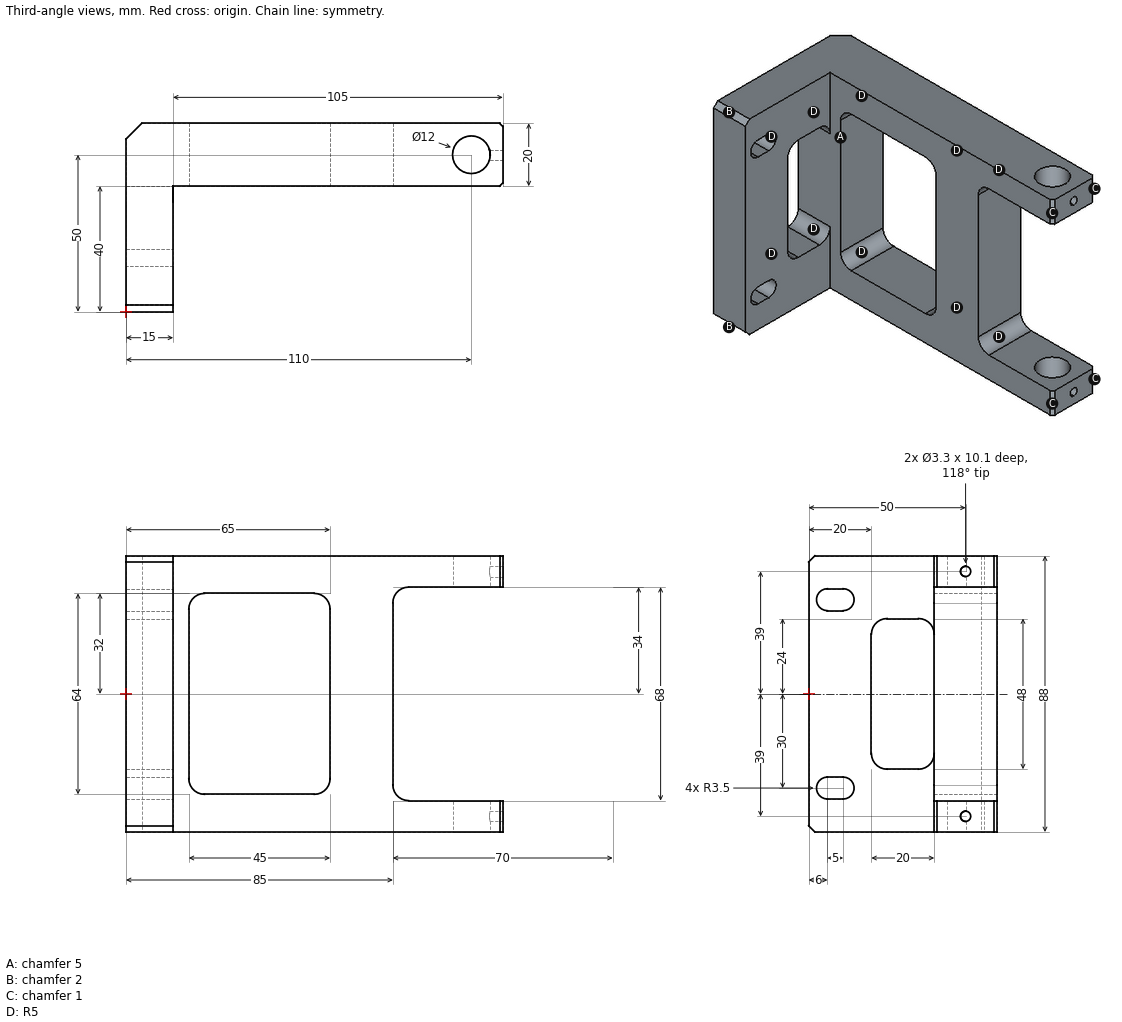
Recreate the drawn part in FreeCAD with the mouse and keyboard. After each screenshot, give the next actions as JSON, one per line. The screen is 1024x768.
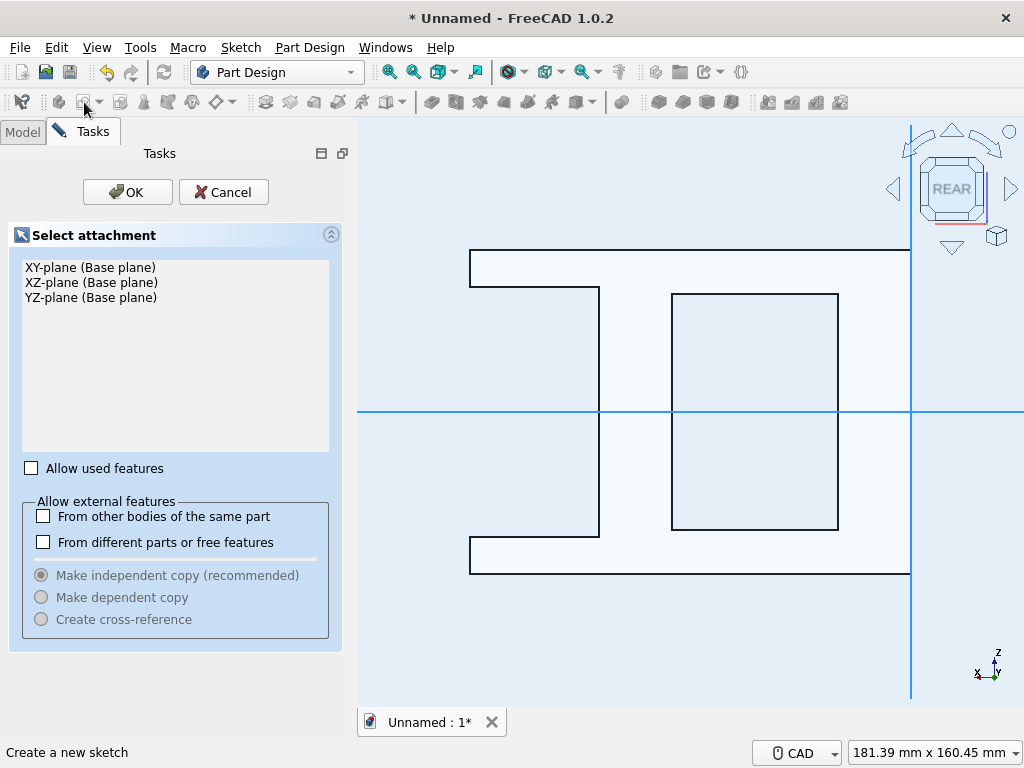
{"action": "left_click", "coordinate": [82, 298]}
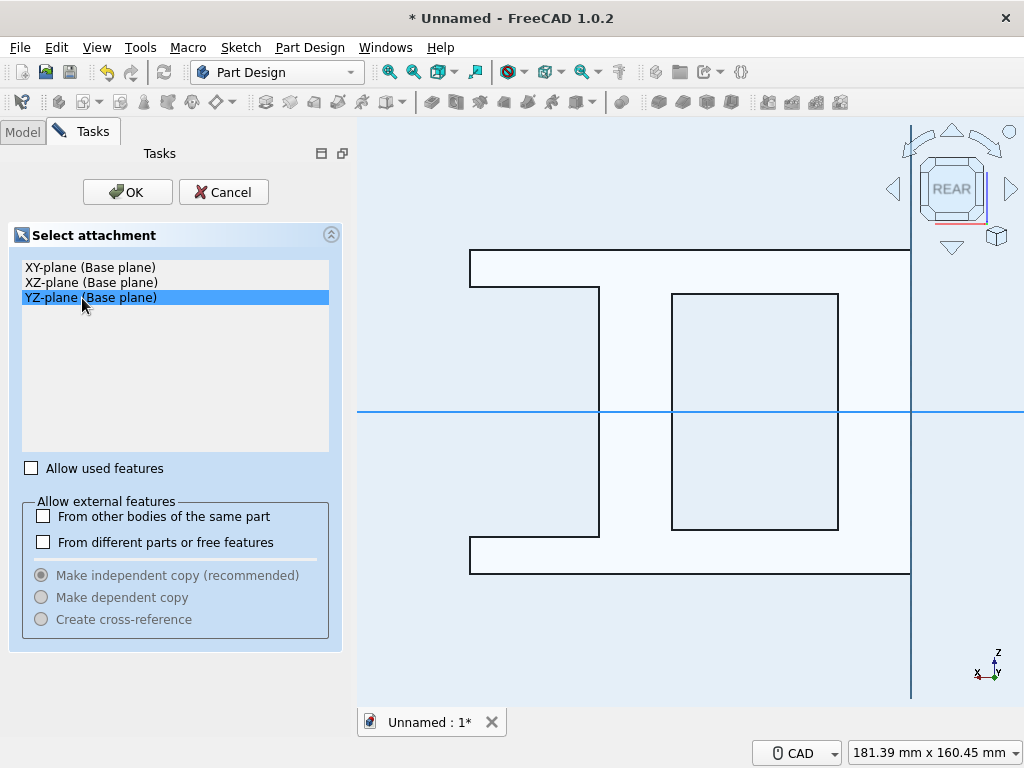
{"action": "left_click", "coordinate": [128, 192]}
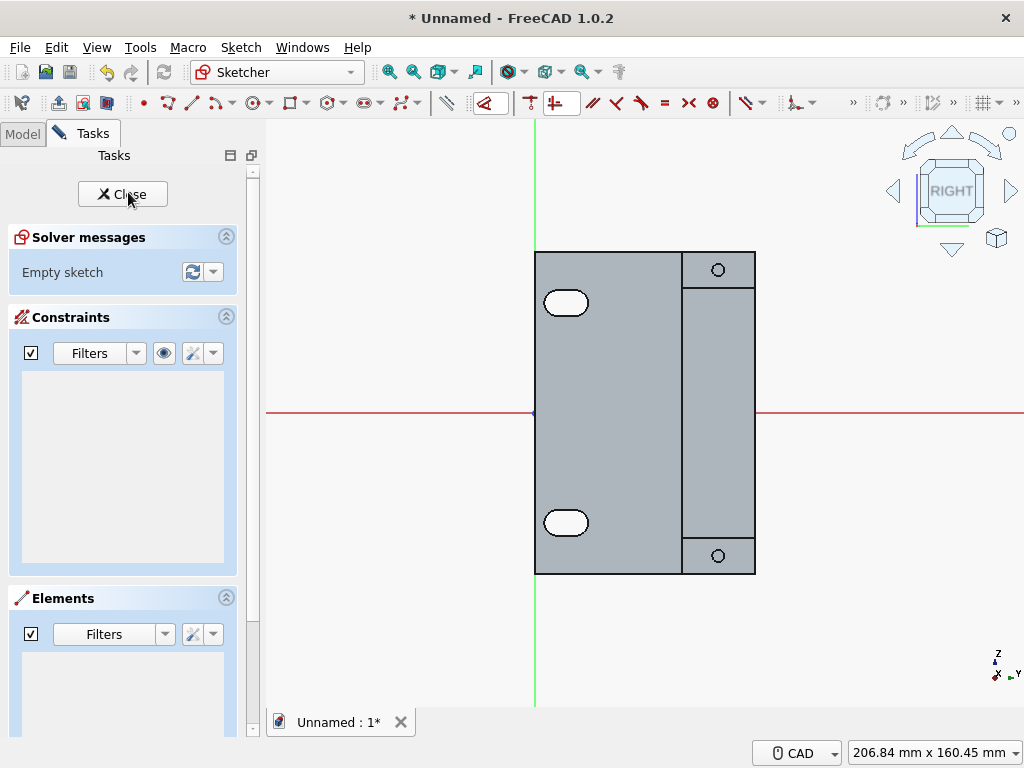
{"action": "key", "text": "q s"}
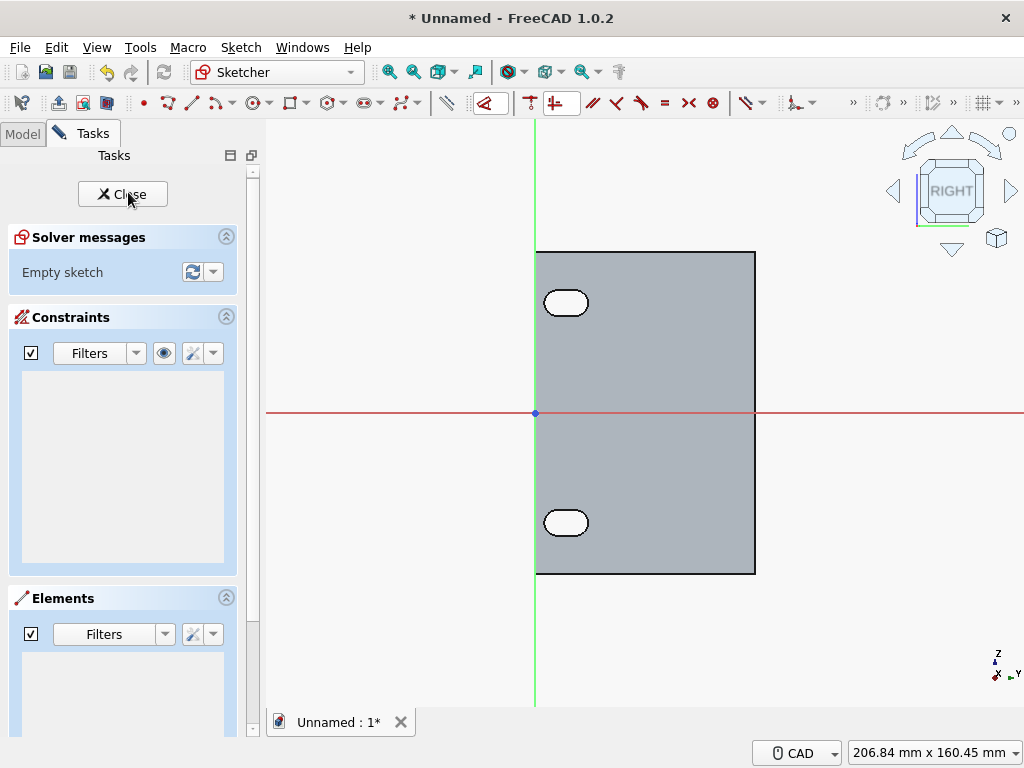
{"action": "scroll", "coordinate": [634, 413], "scroll_direction": "up", "scroll_amount": 4}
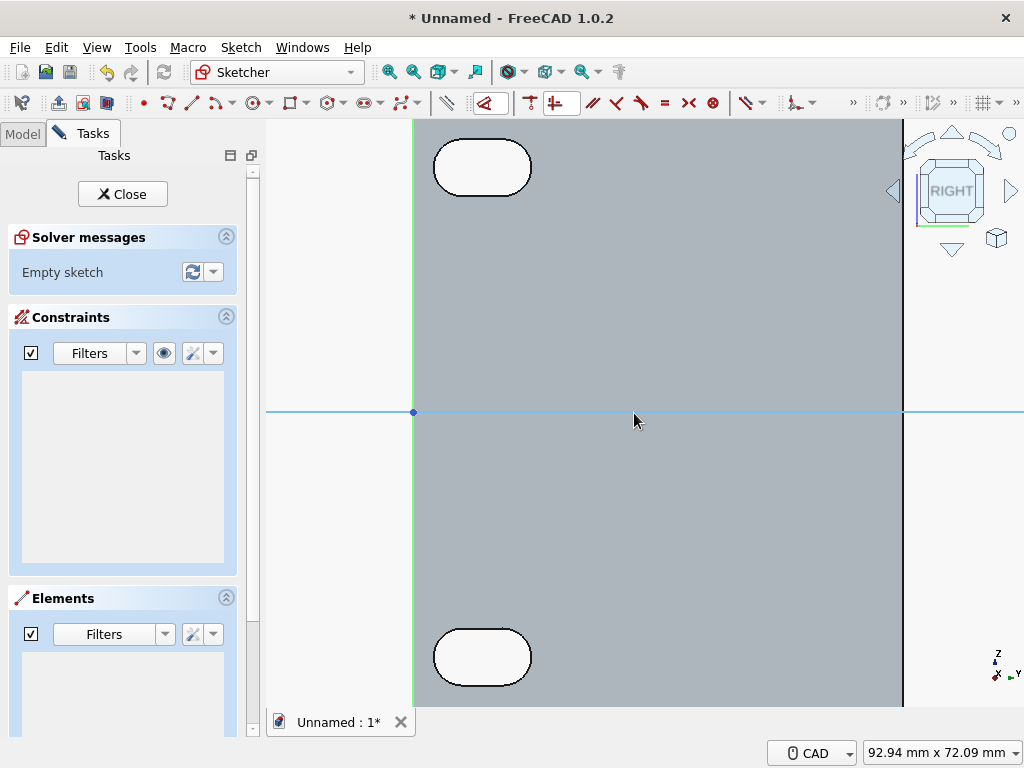
{"action": "left_click", "coordinate": [290, 104]}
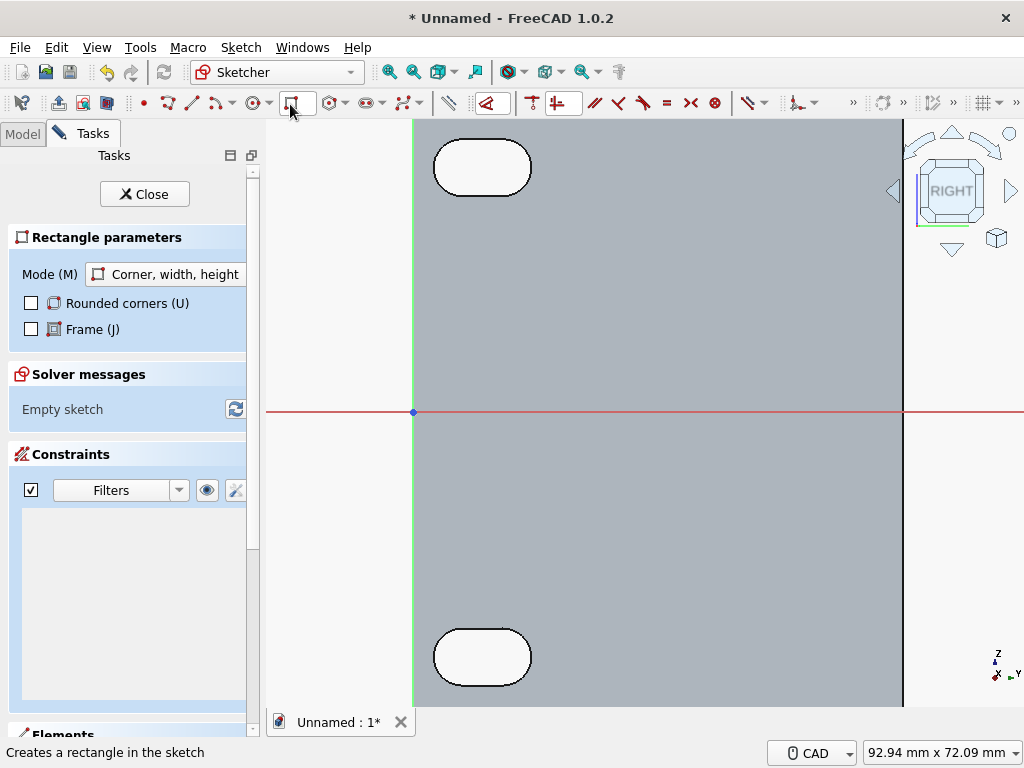
{"action": "left_click", "coordinate": [576, 217]}
{"action": "mouse_move", "coordinate": [739, 608]}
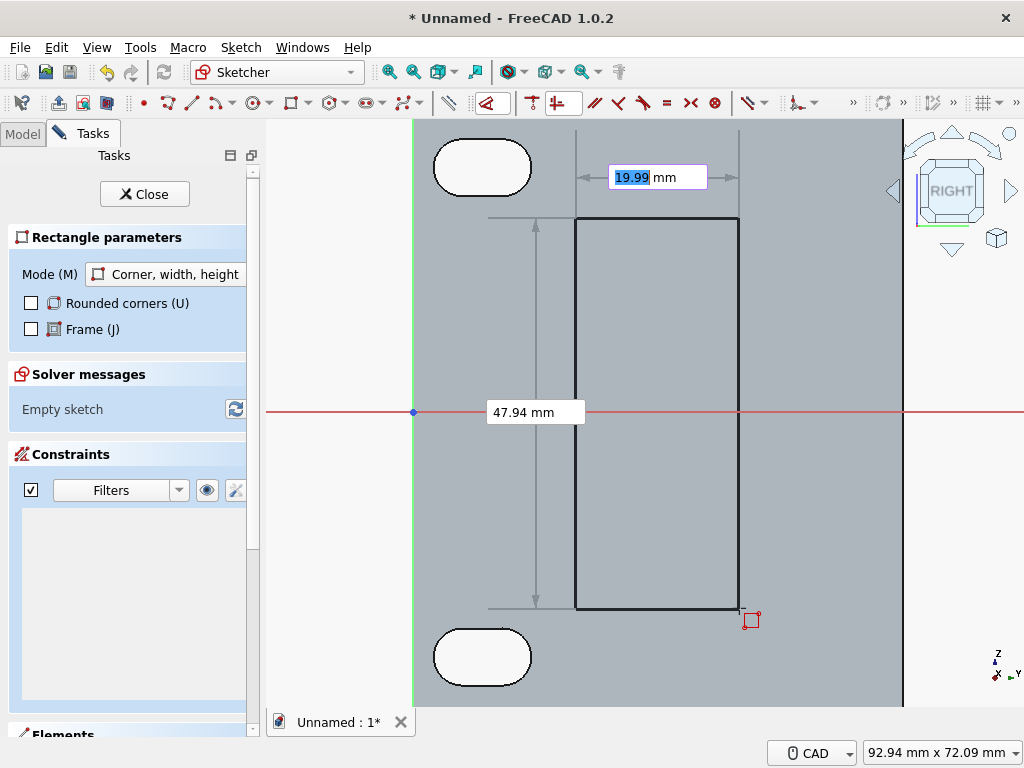
{"action": "type", "text": "20"}
{"action": "key", "text": "Tab"}
{"action": "type", "text": "48"}
{"action": "key", "text": "Return"}
{"action": "key", "text": "Escape"}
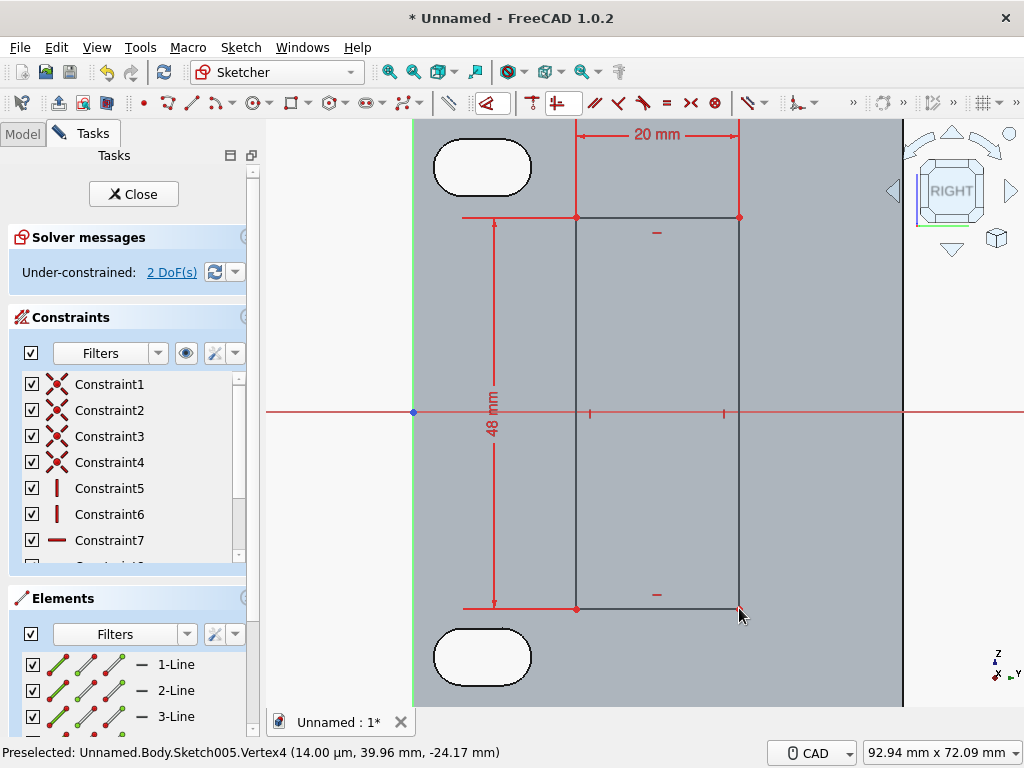
{"action": "left_click", "coordinate": [576, 218]}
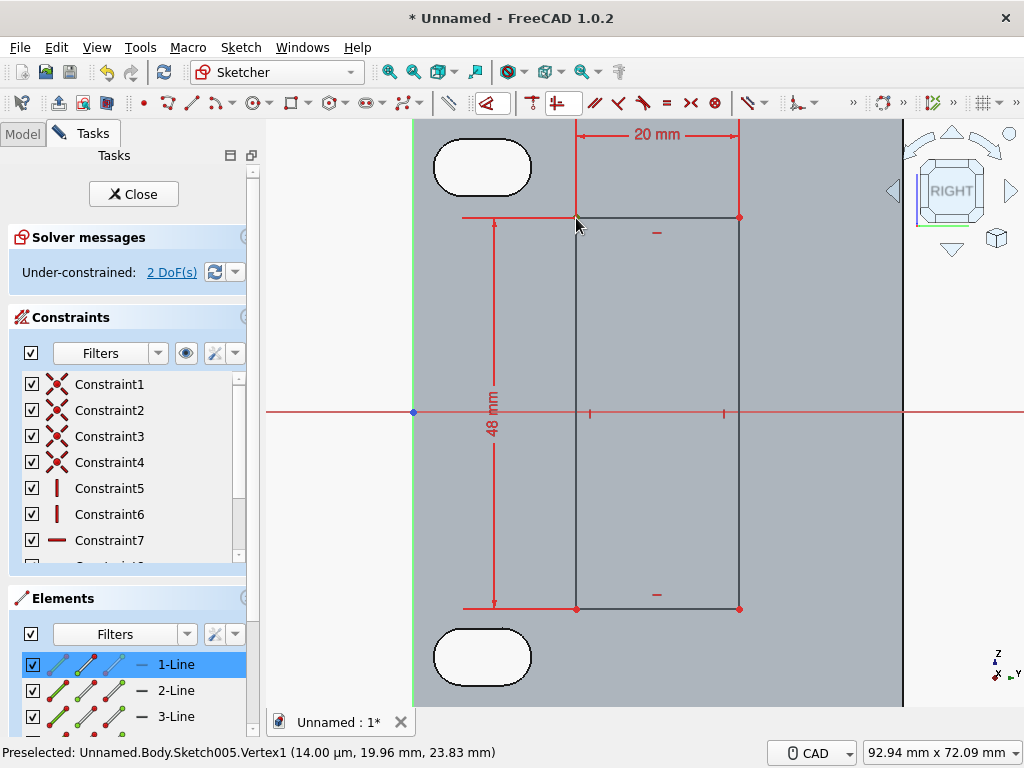
{"action": "key", "text": "l"}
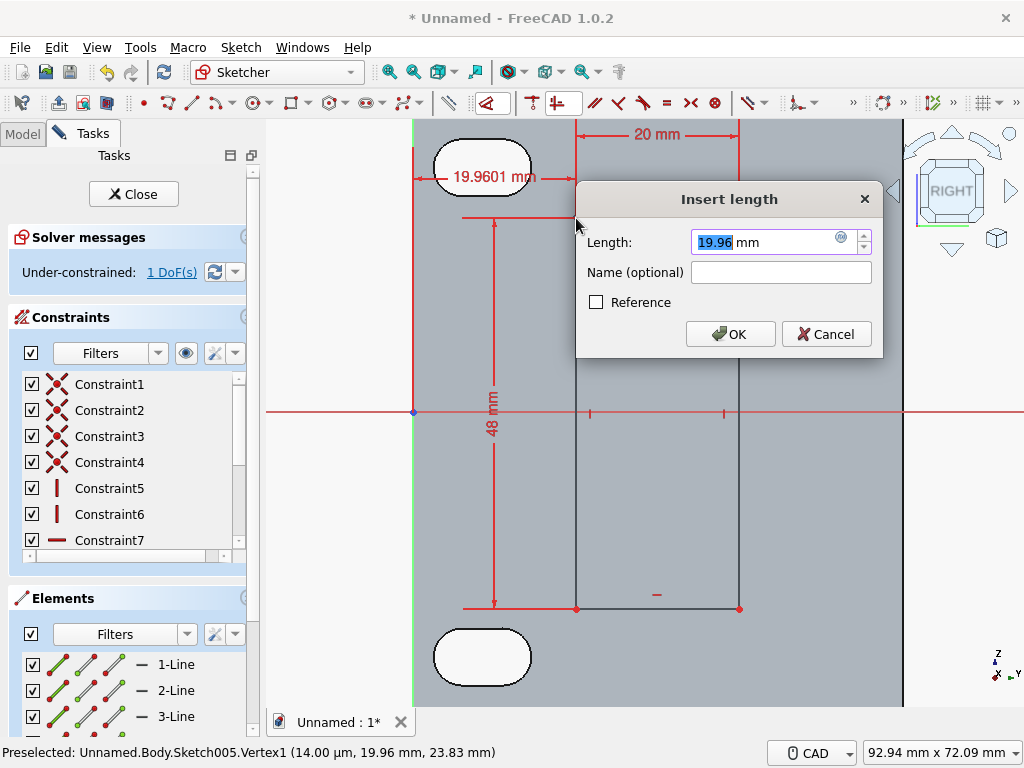
{"action": "type", "text": "20"}
{"action": "key", "text": "Return"}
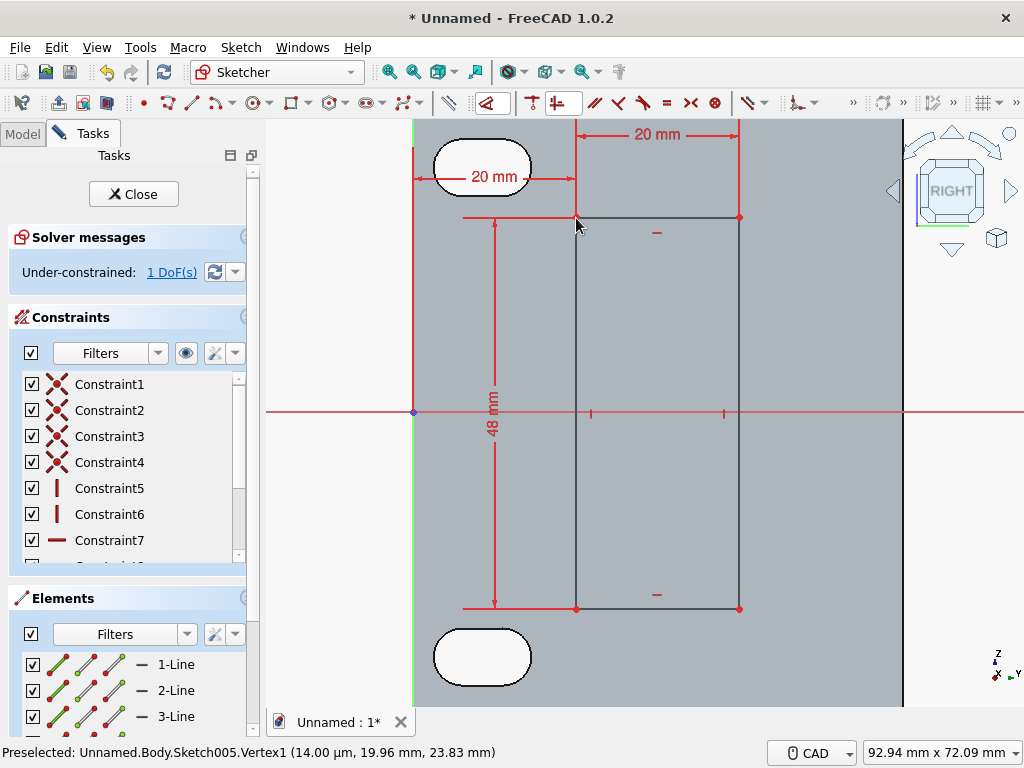
{"action": "left_click", "coordinate": [576, 218]}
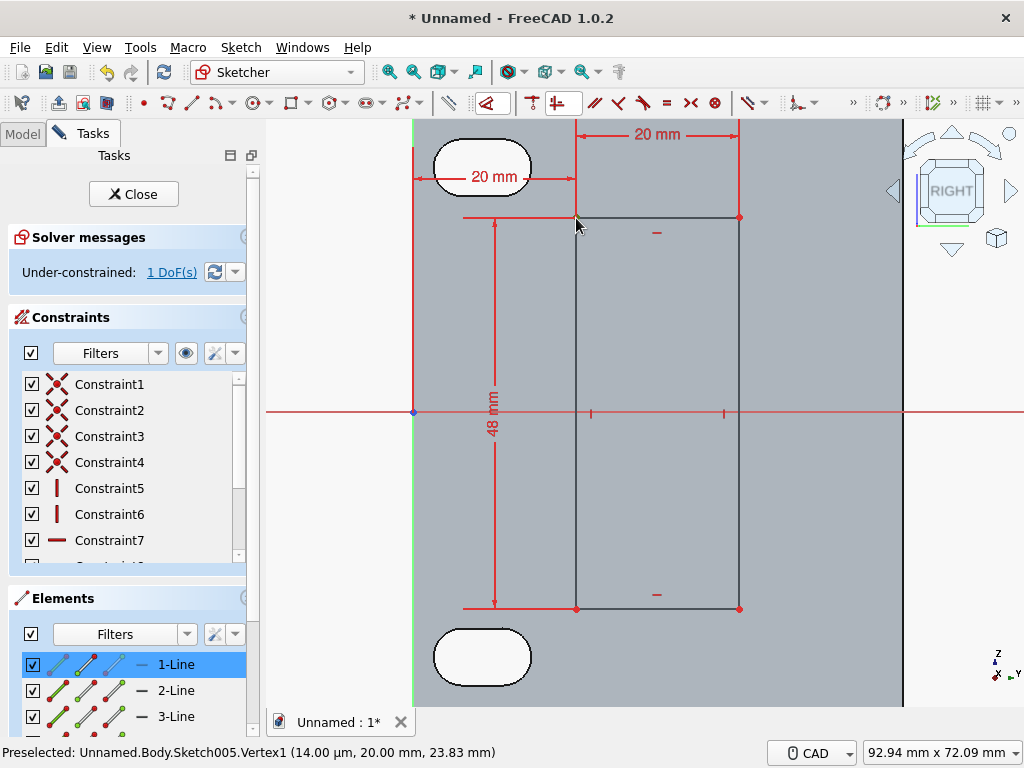
{"action": "key", "text": "i"}